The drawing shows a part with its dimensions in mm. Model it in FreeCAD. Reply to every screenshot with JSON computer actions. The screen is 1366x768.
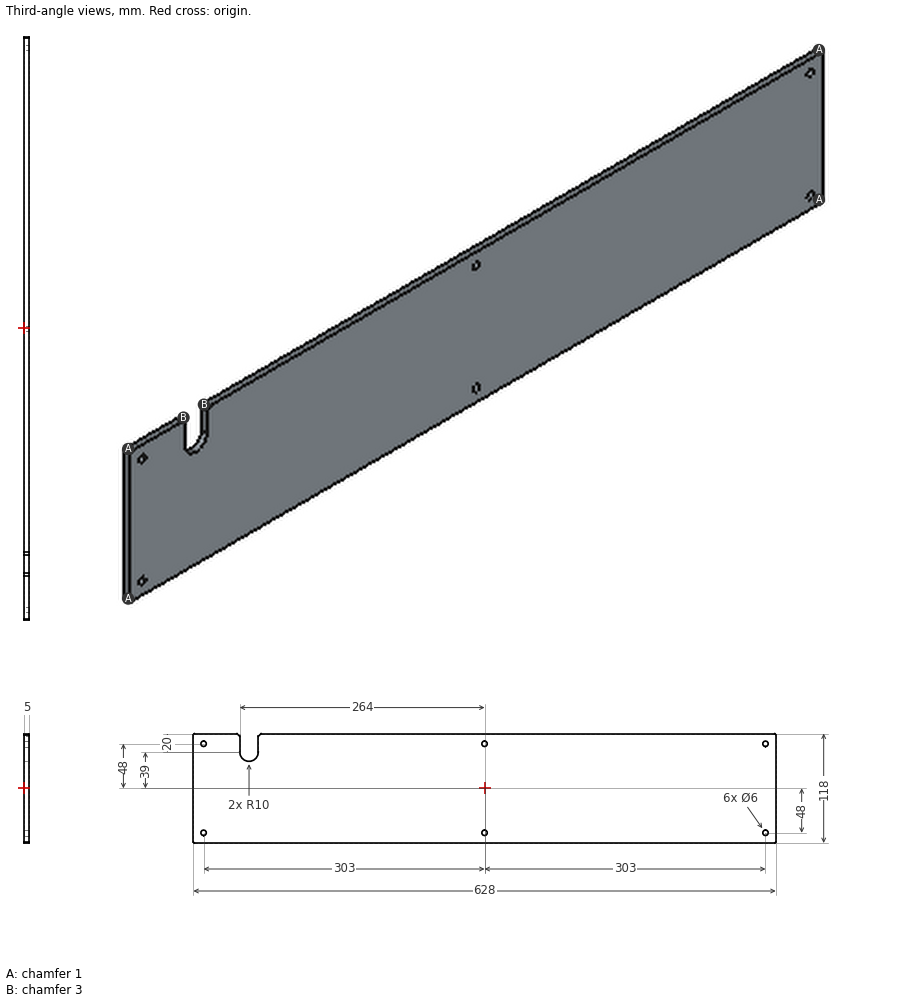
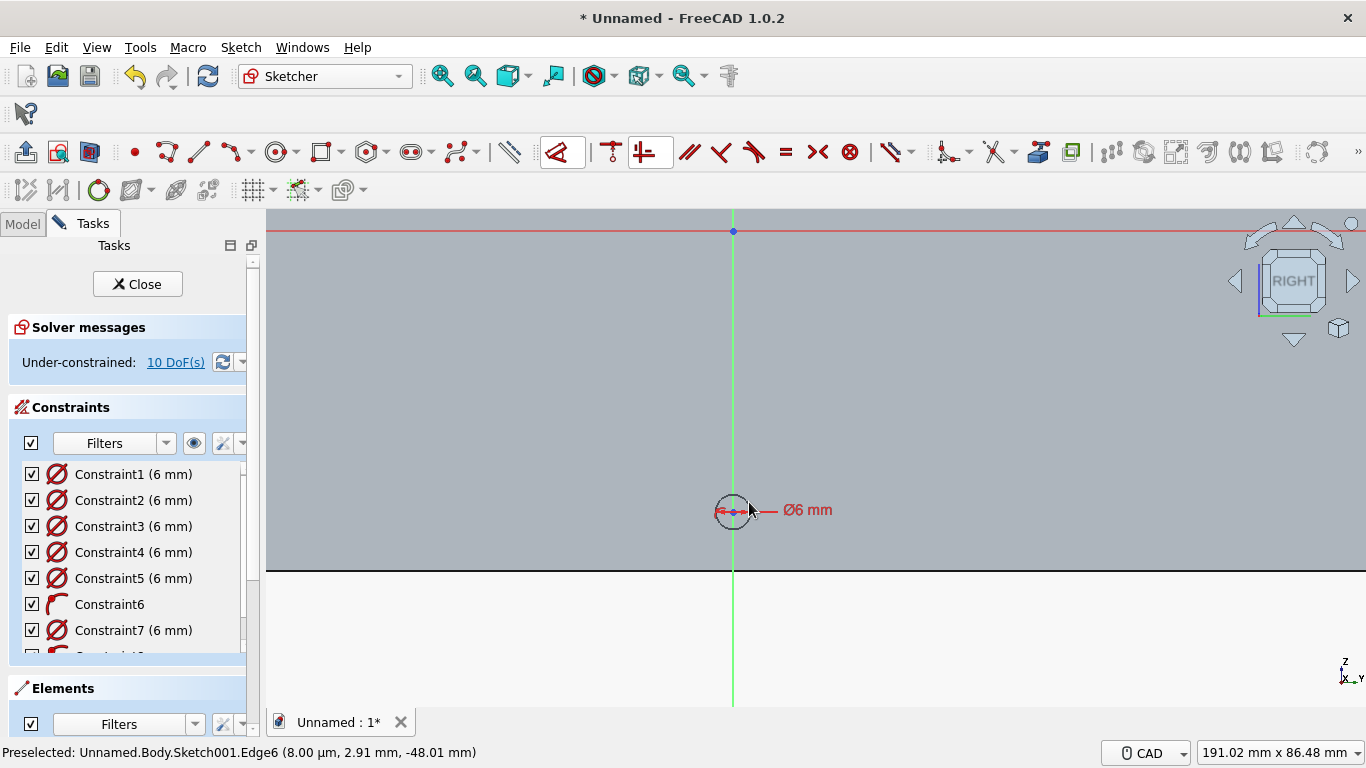
{"action": "scroll", "coordinate": [750, 503], "scroll_direction": "down", "scroll_amount": 9}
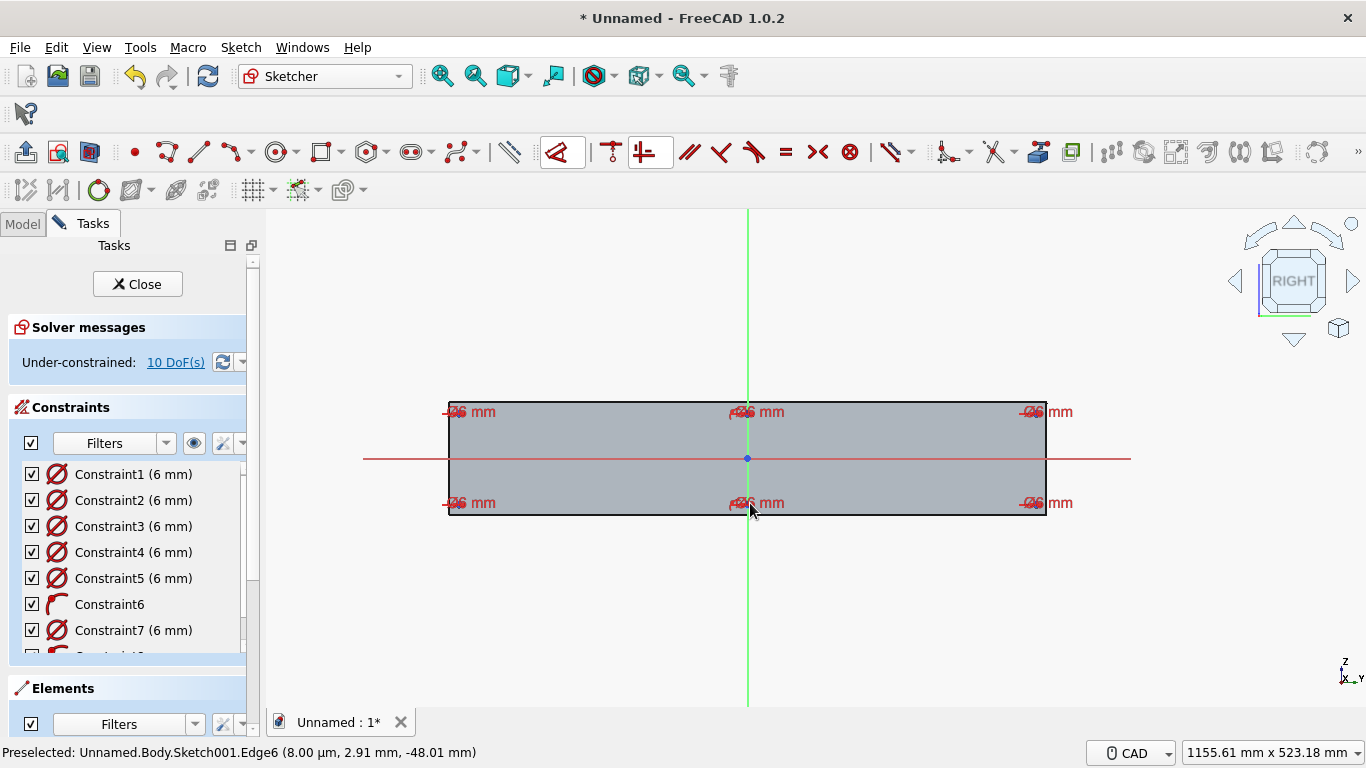
{"action": "left_click", "coordinate": [1036, 505]}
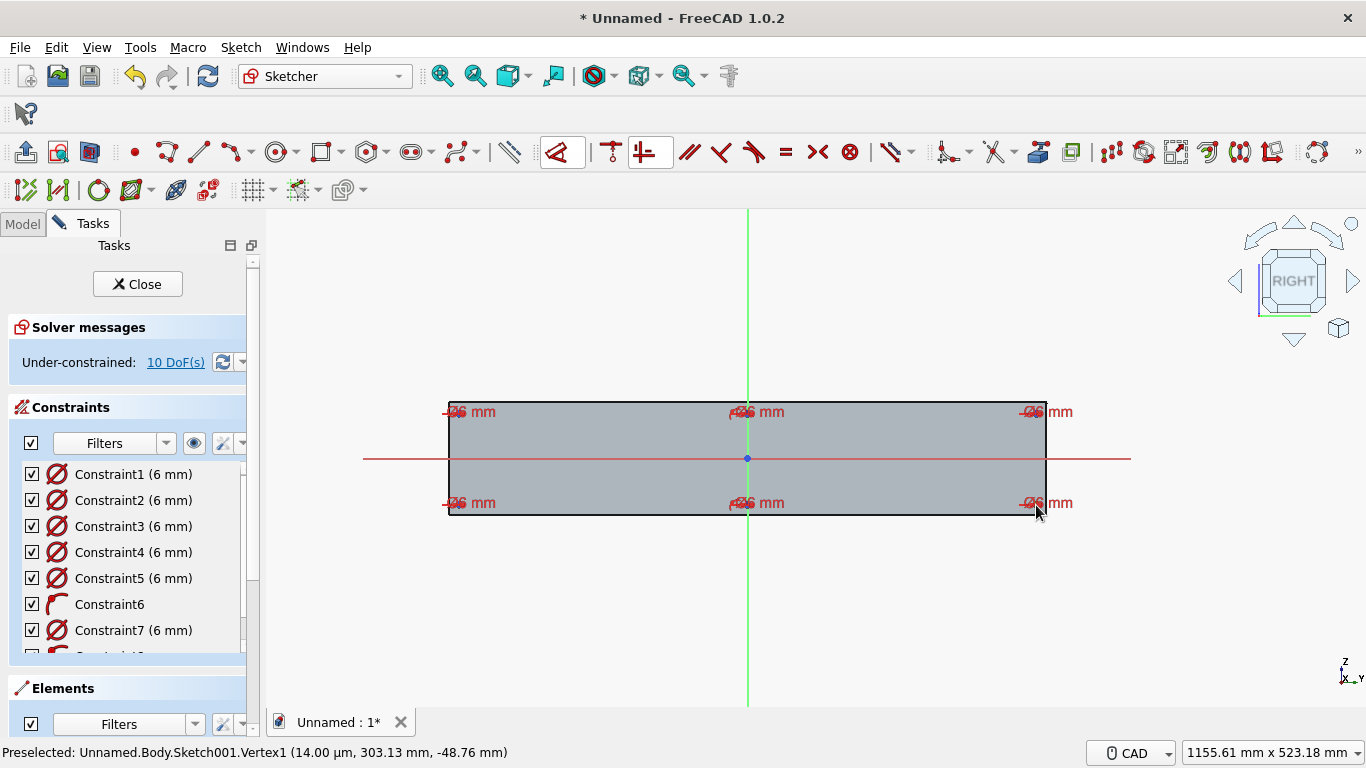
{"action": "left_click", "coordinate": [459, 505]}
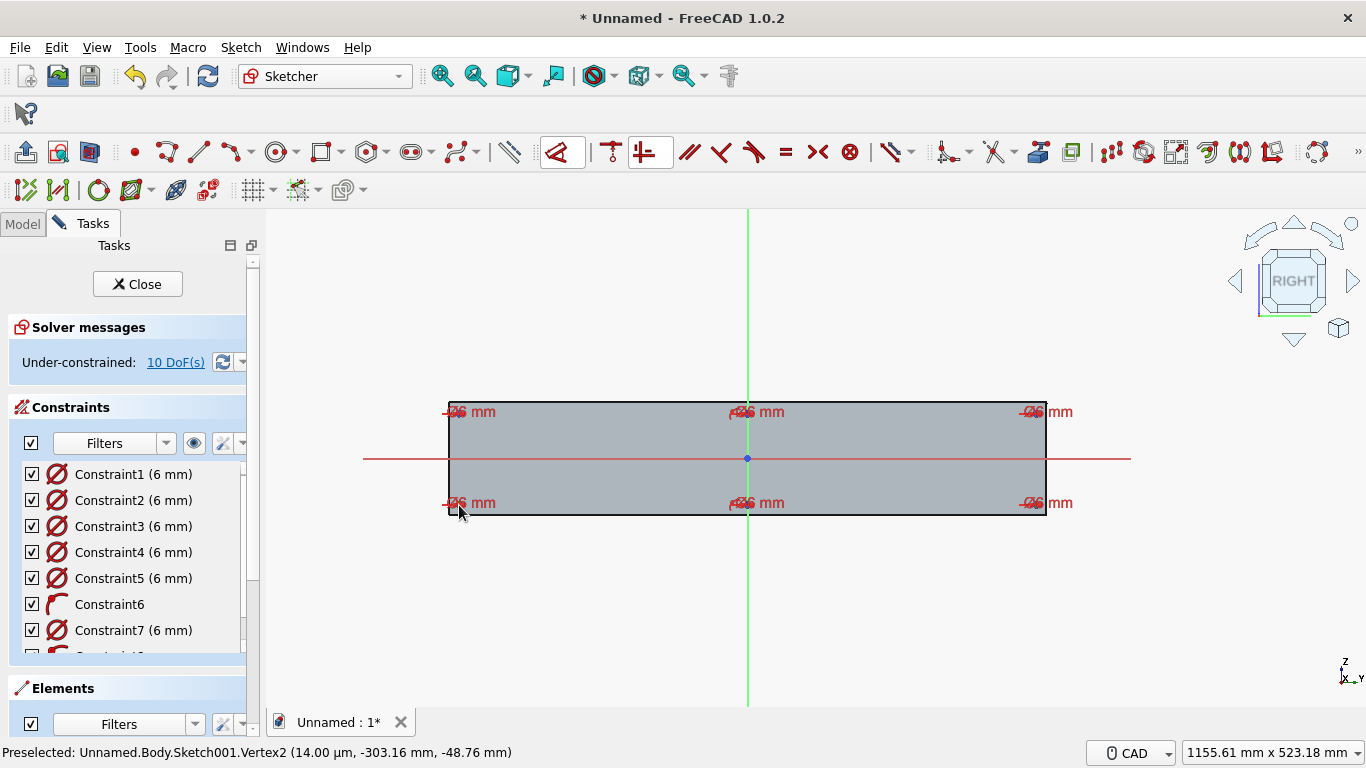
{"action": "key", "text": "h"}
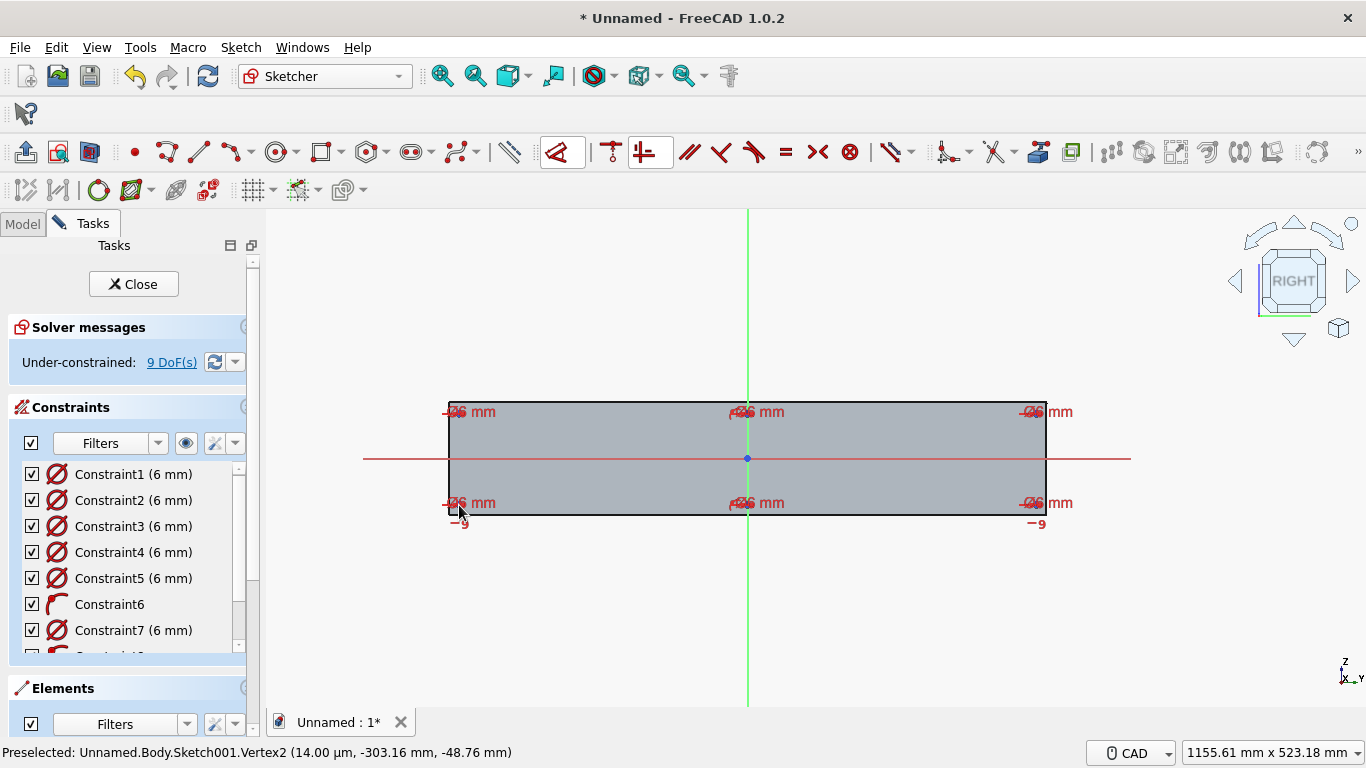
{"action": "left_click", "coordinate": [459, 505]}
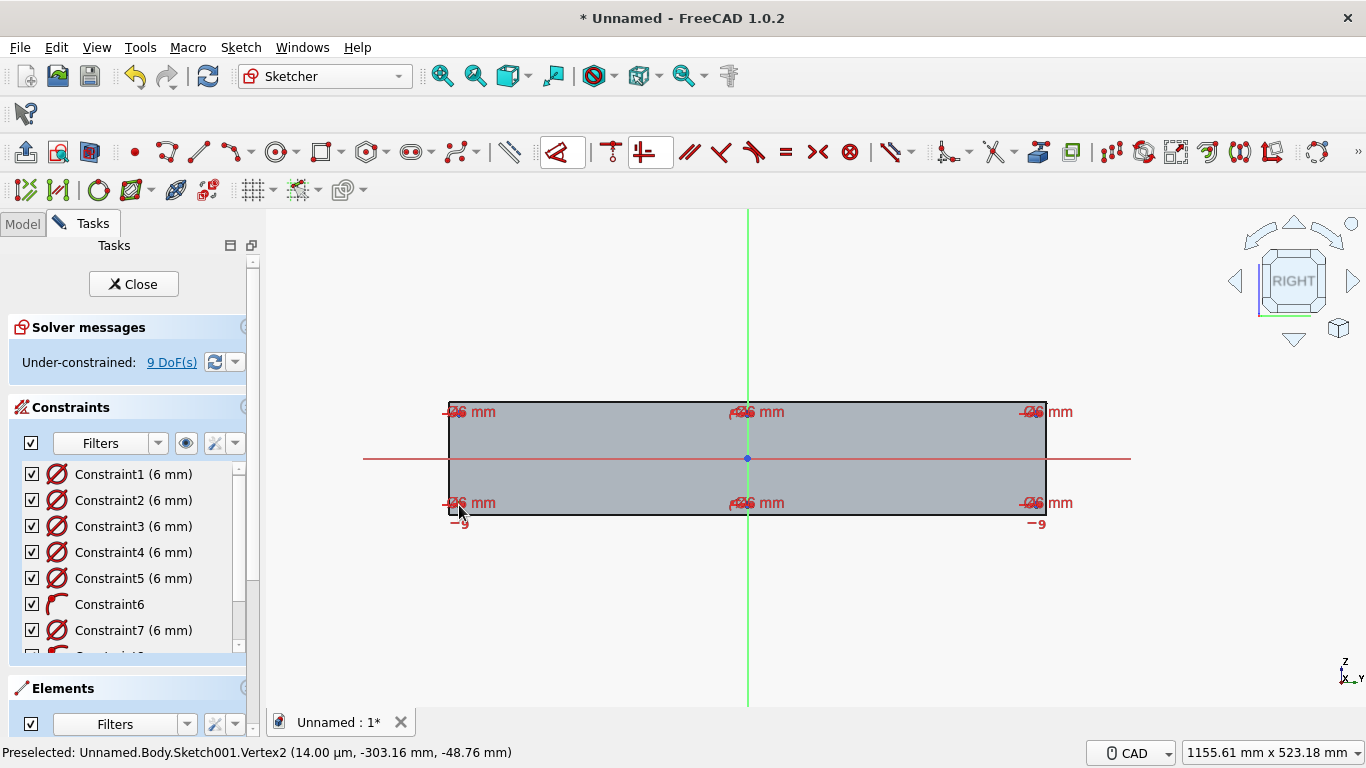
{"action": "left_click", "coordinate": [459, 414]}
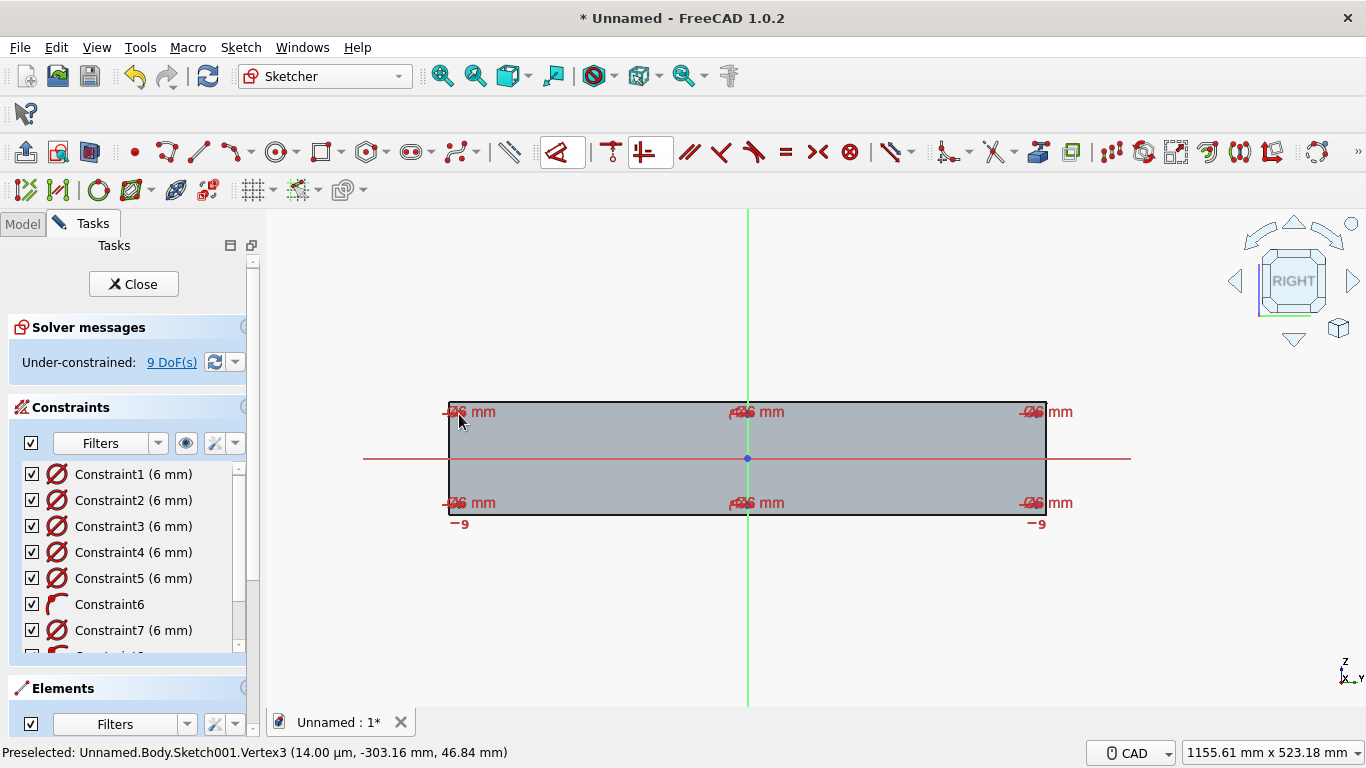
{"action": "key", "text": "v"}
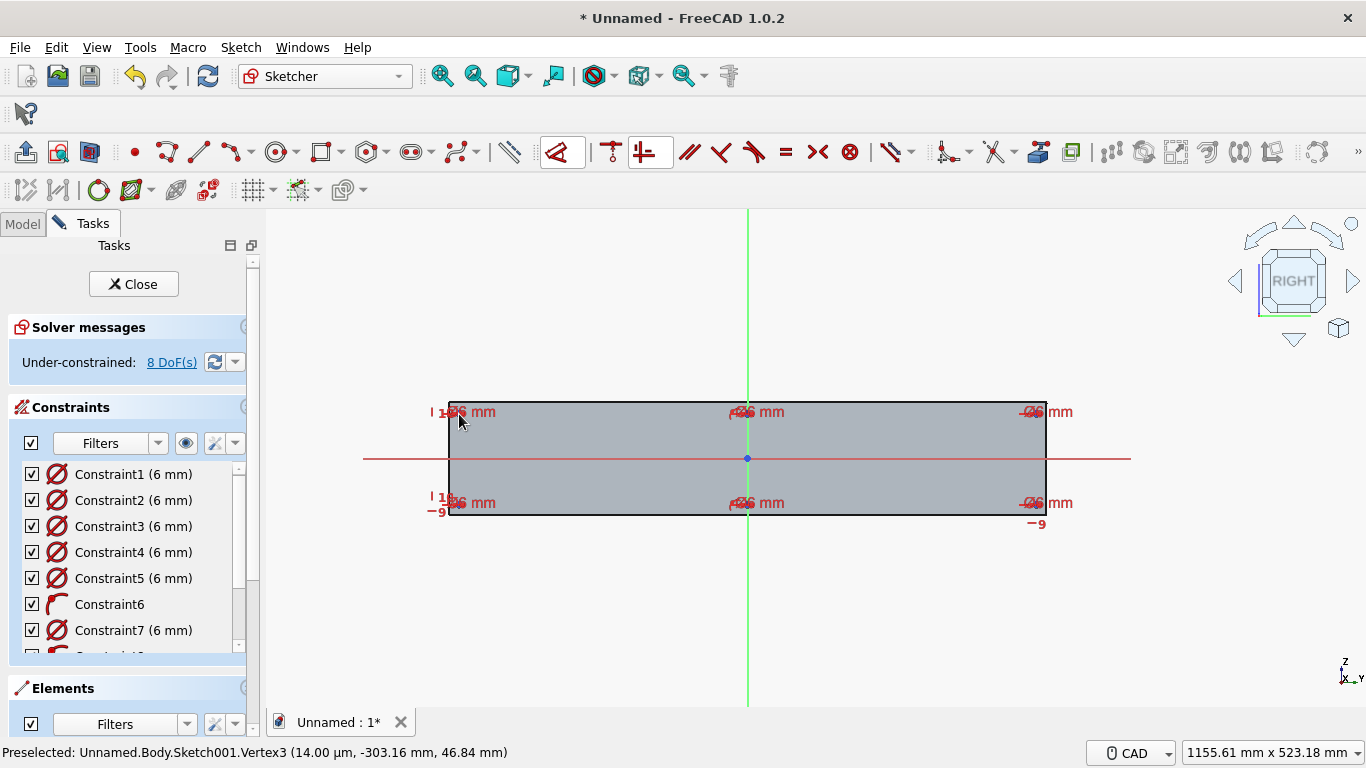
{"action": "left_click", "coordinate": [1036, 505]}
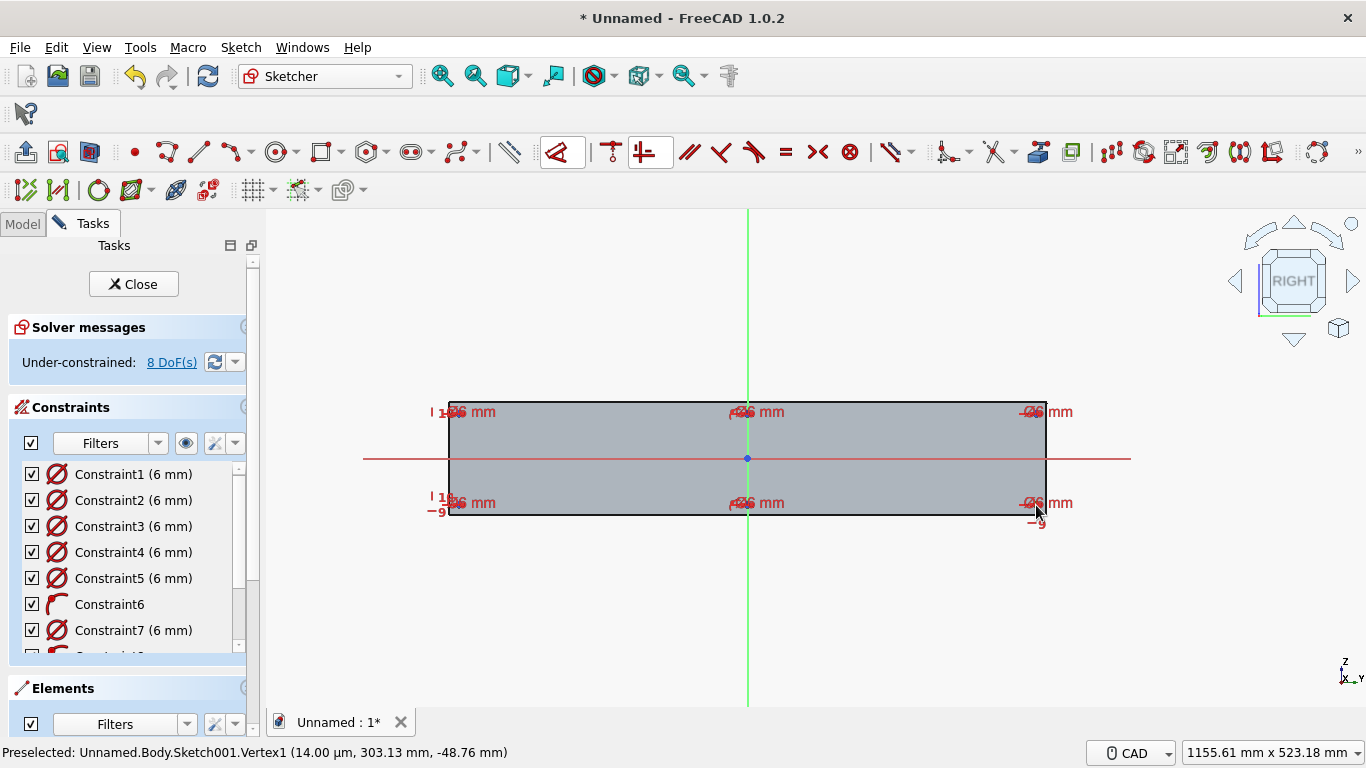
{"action": "left_click", "coordinate": [1036, 414]}